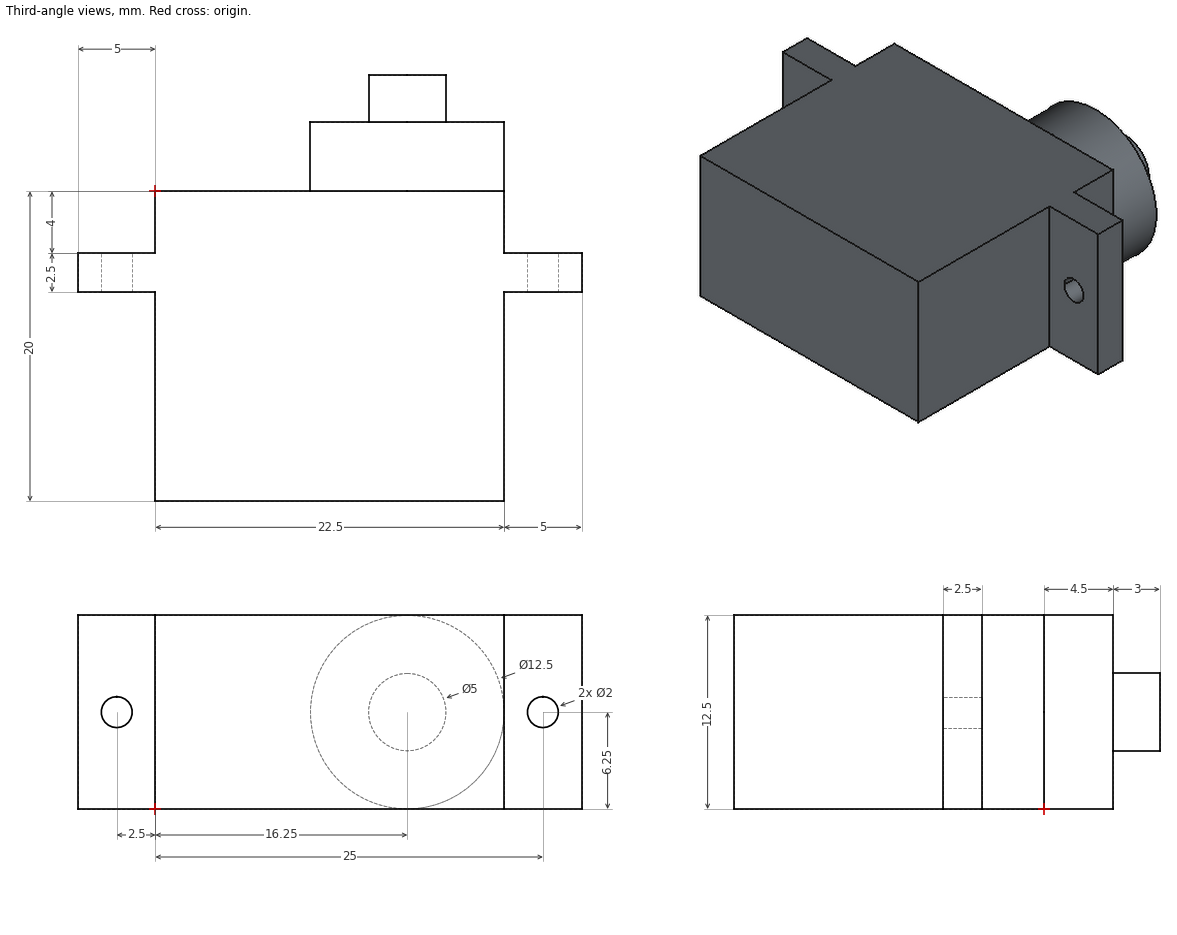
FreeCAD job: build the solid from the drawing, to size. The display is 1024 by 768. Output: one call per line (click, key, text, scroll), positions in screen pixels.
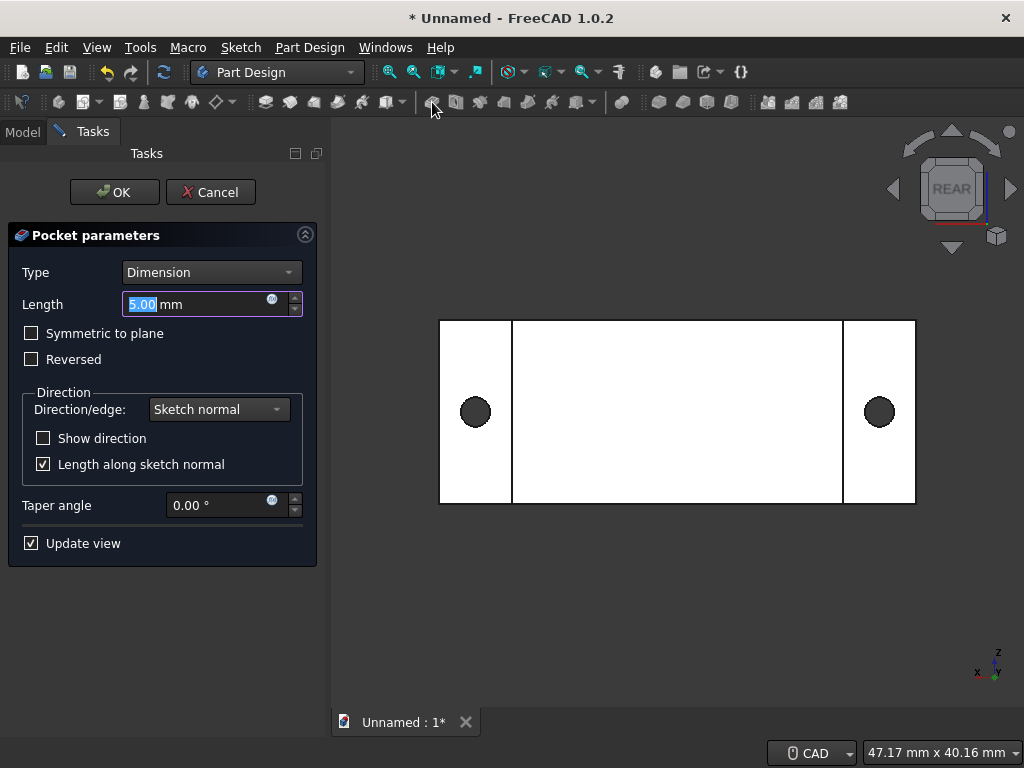
text(2.5)
key(Tab)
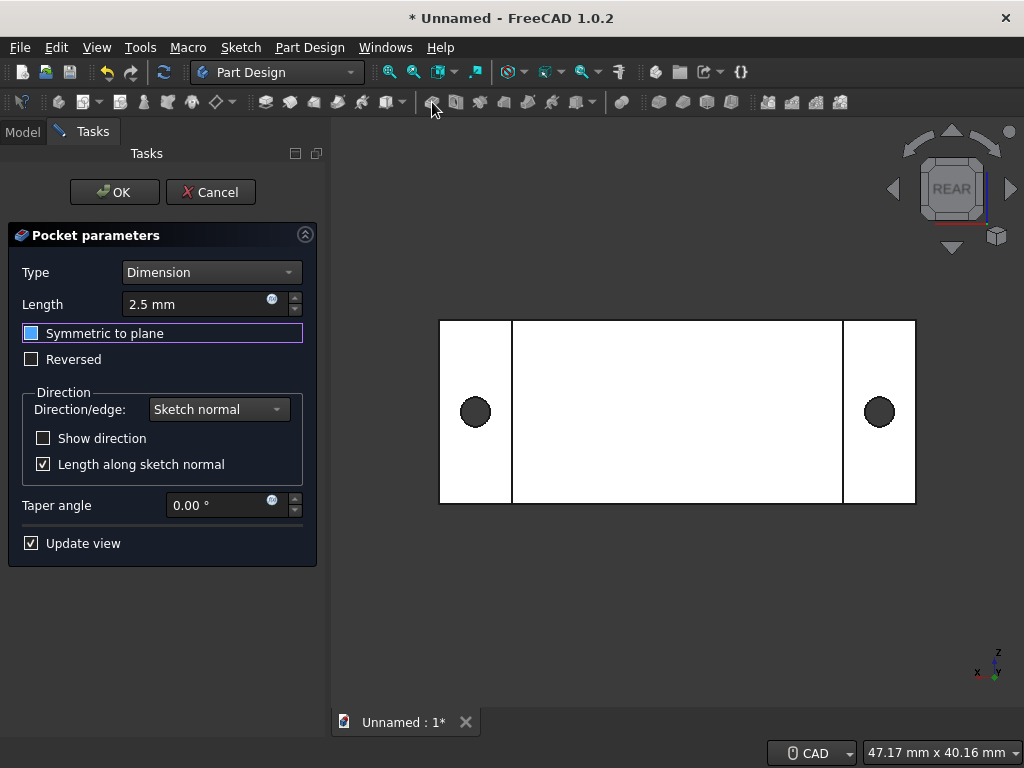
click(115, 192)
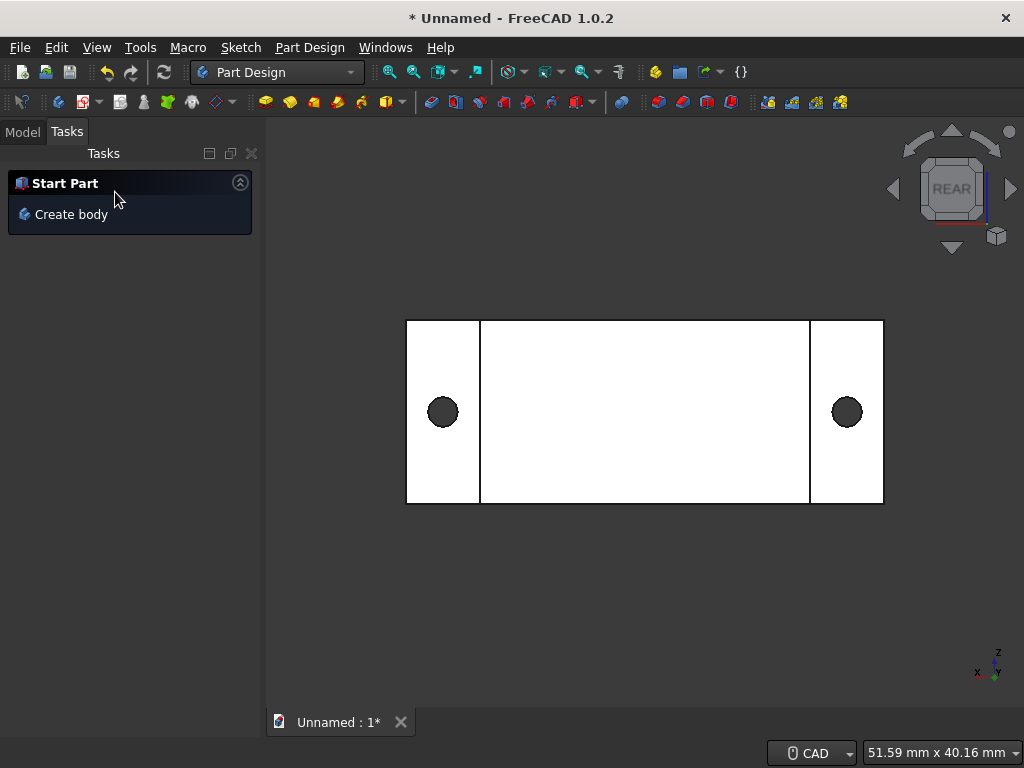
click(598, 411)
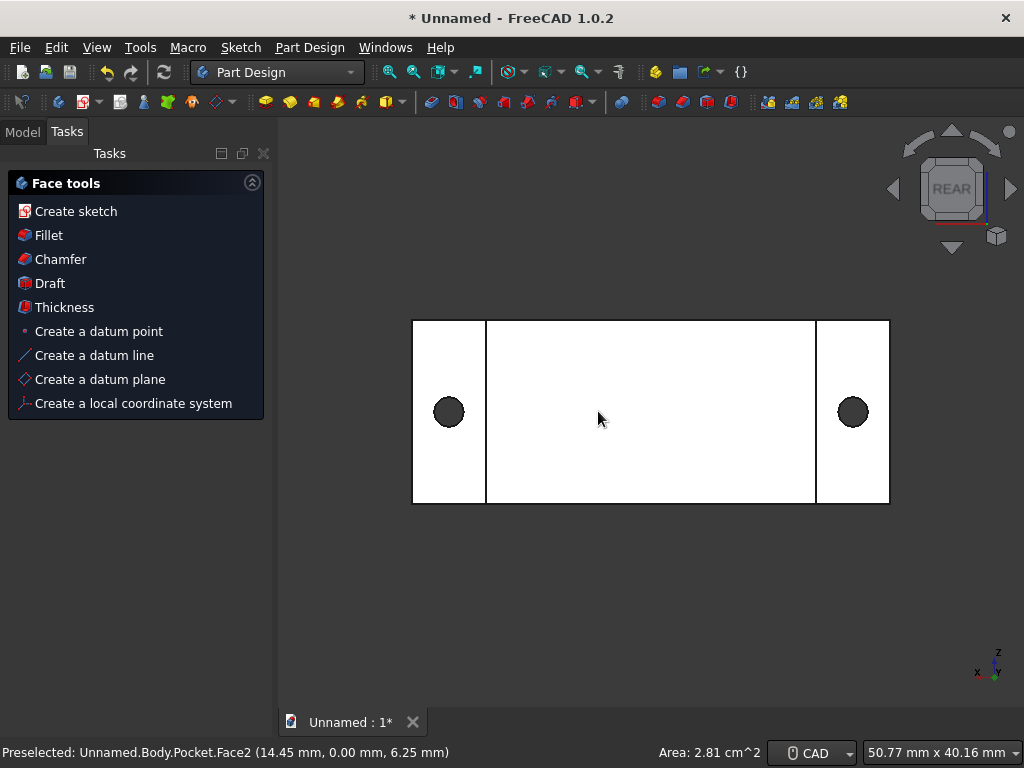
click(84, 102)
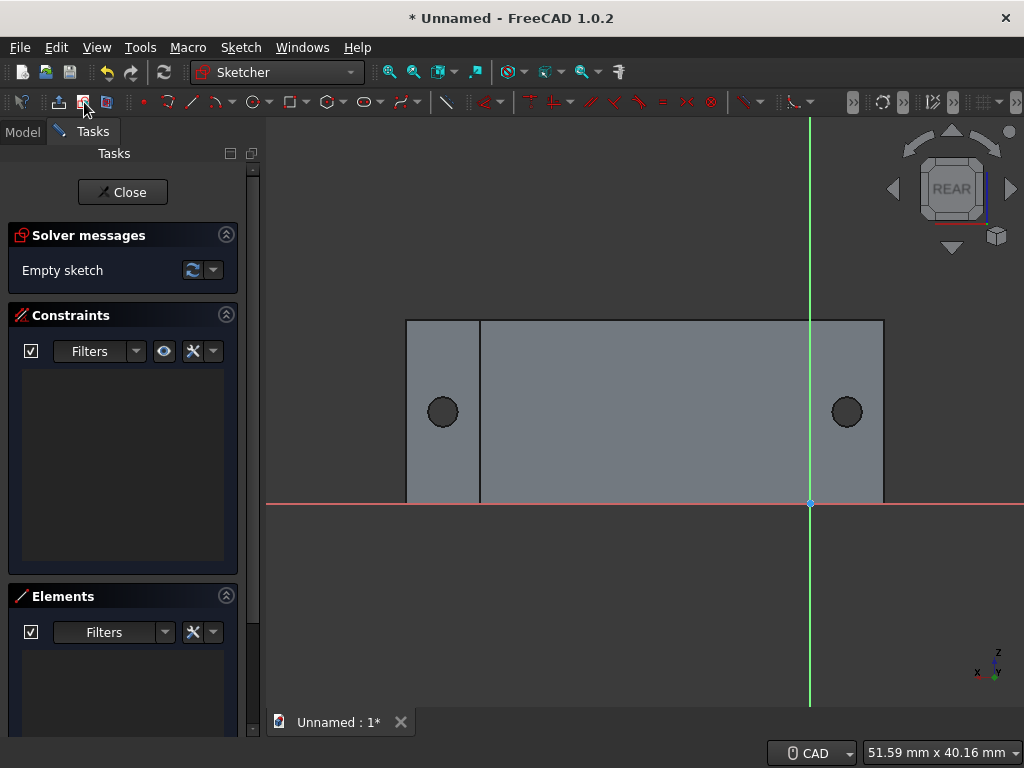
click(254, 102)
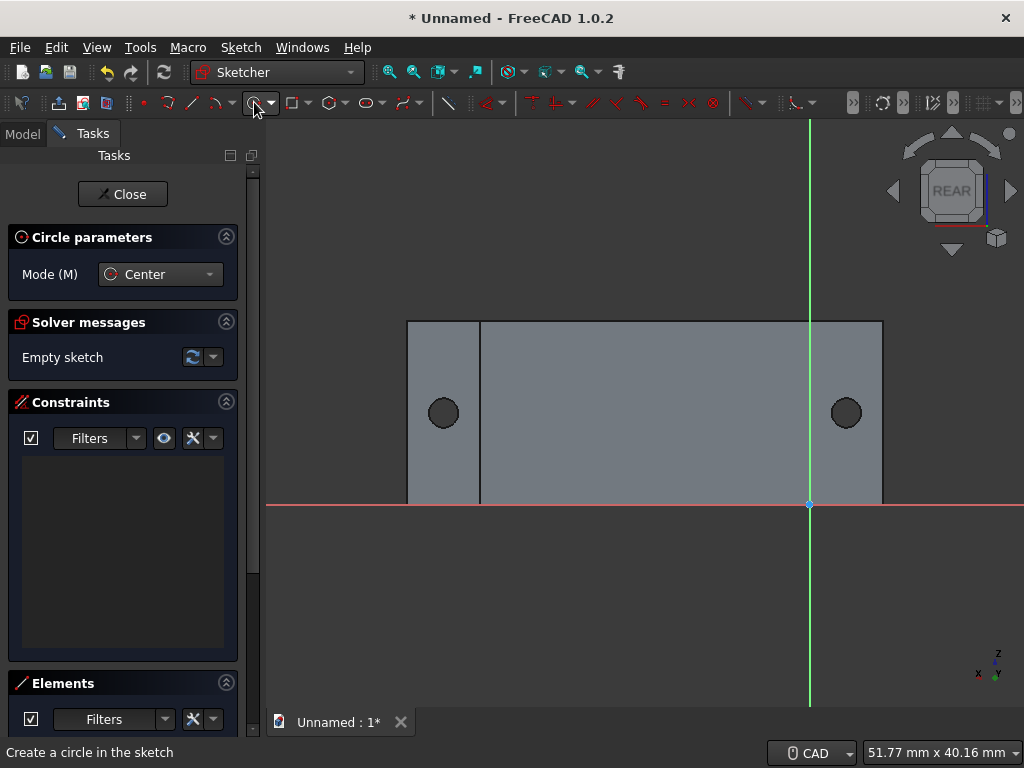
click(572, 413)
move(636, 348)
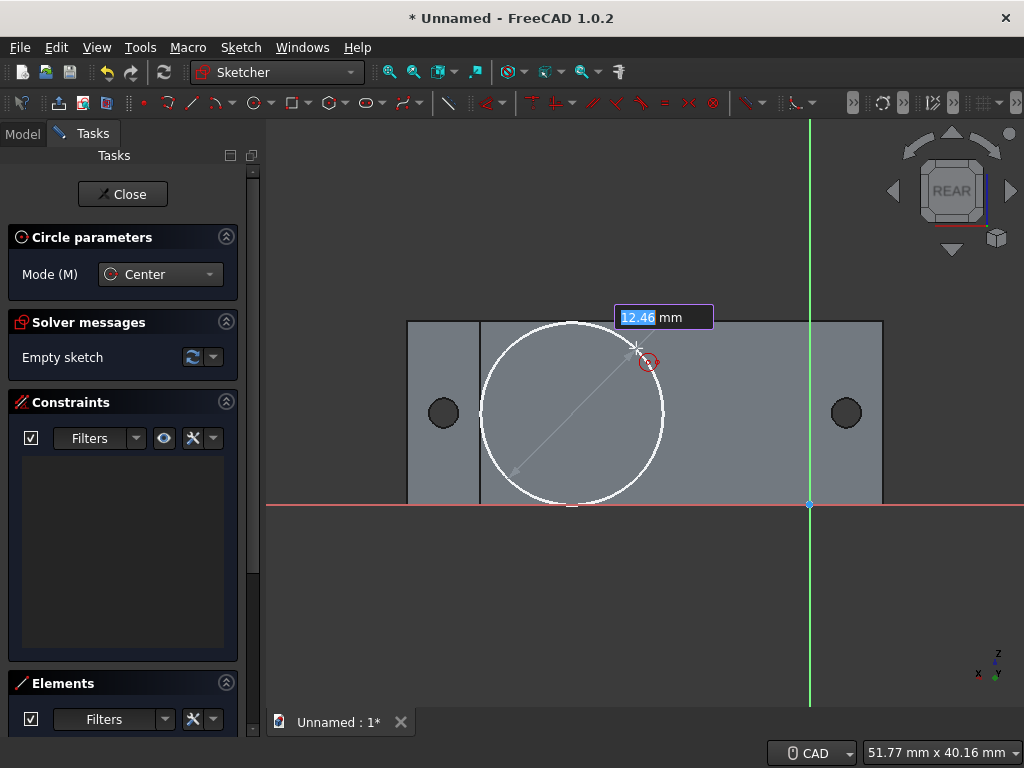
text(12.5)
key(Return)
key(Escape)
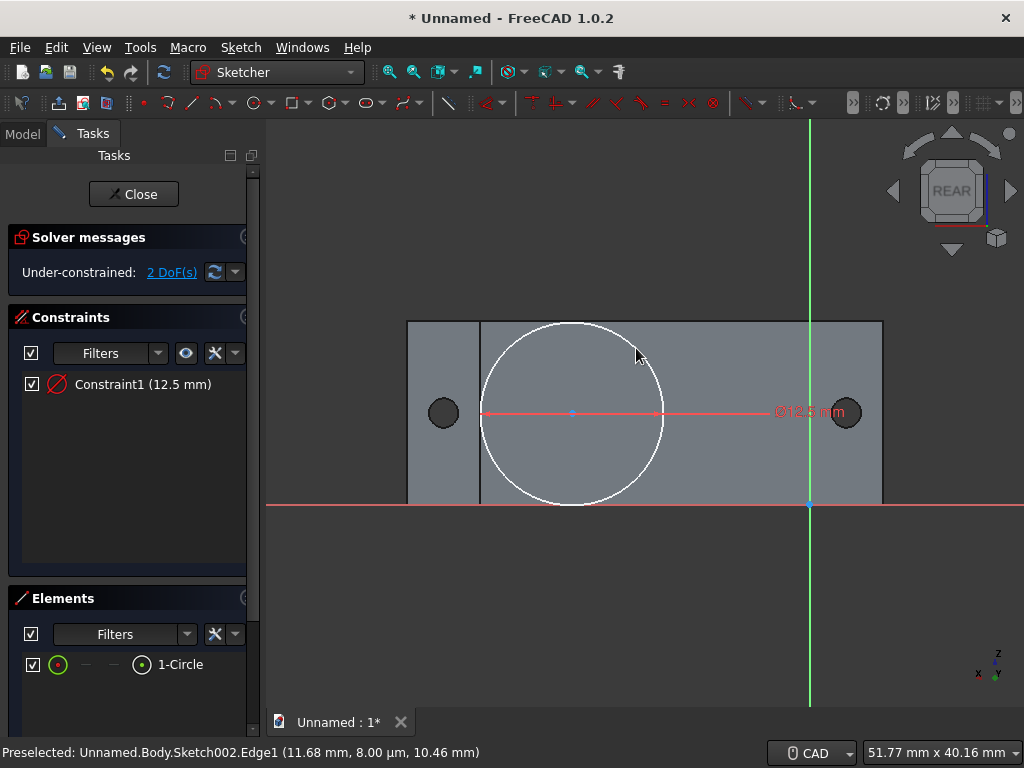
key(d)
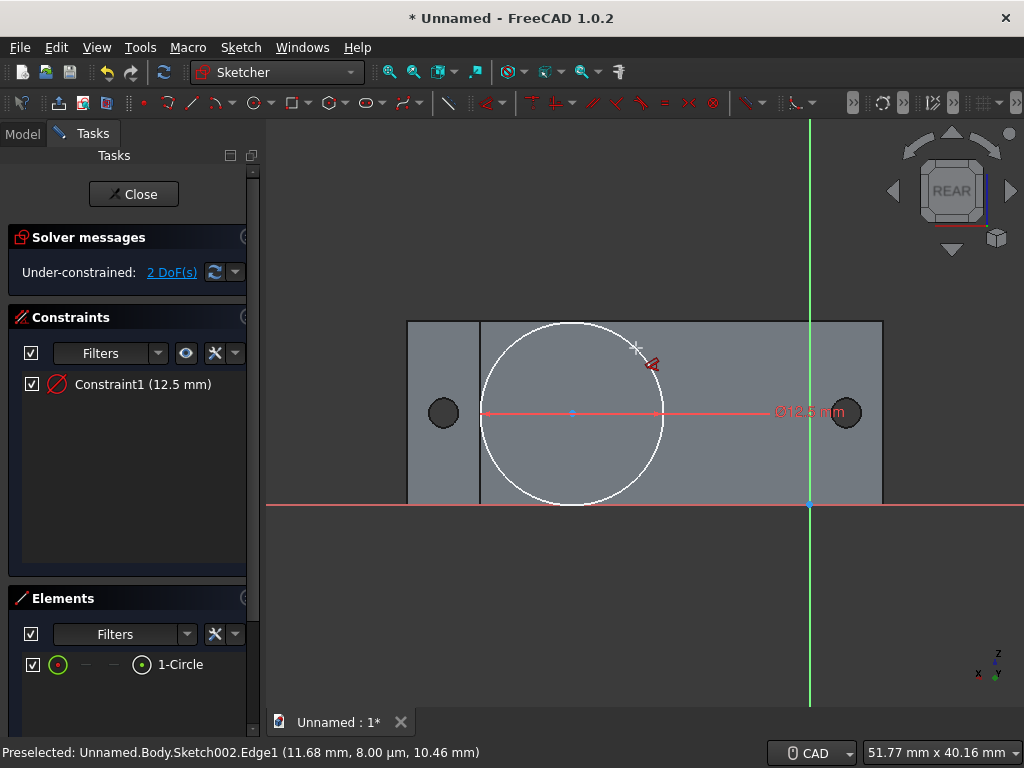
click(572, 414)
click(844, 459)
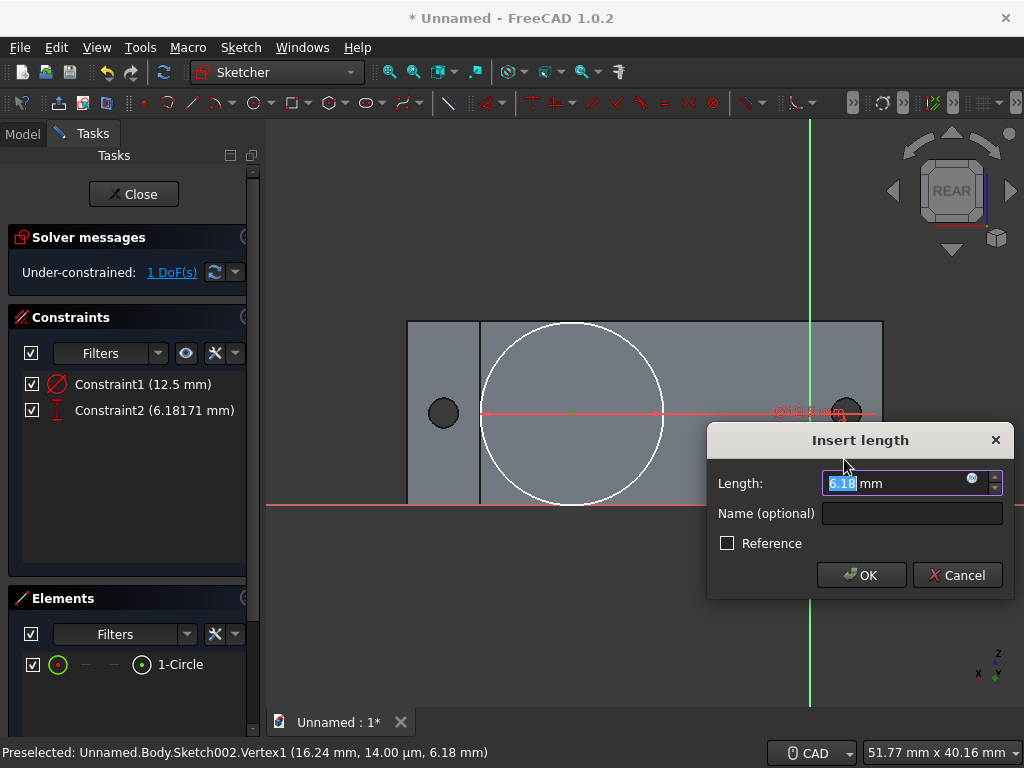
text(6.25)
key(Return)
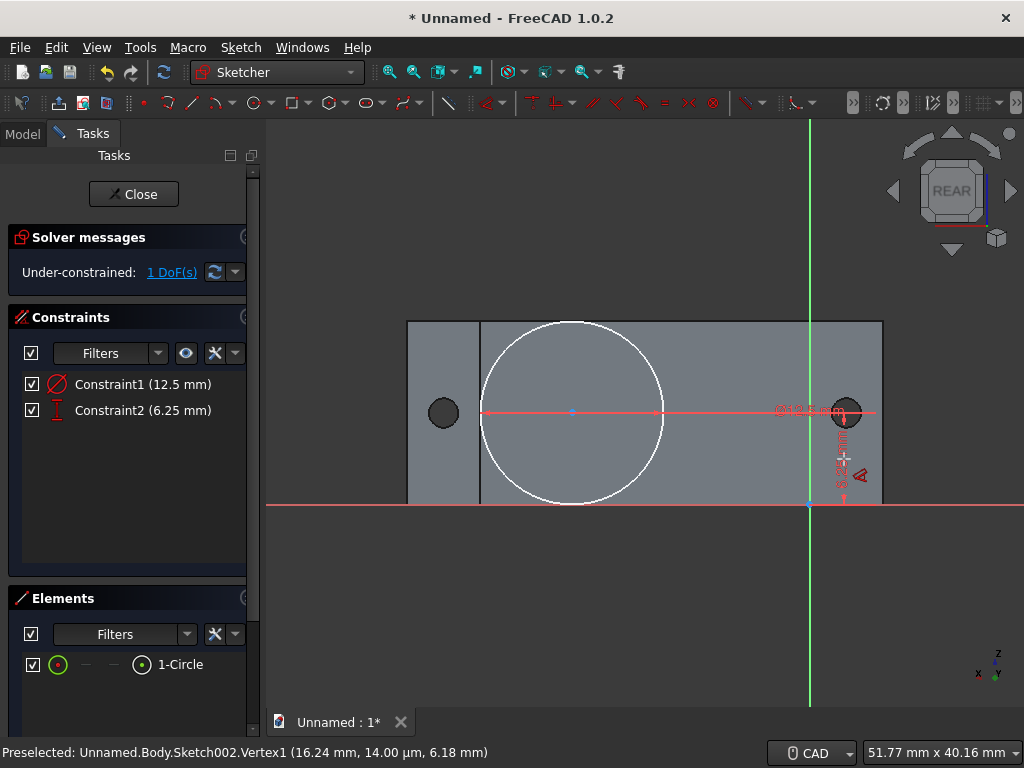
click(572, 413)
click(691, 539)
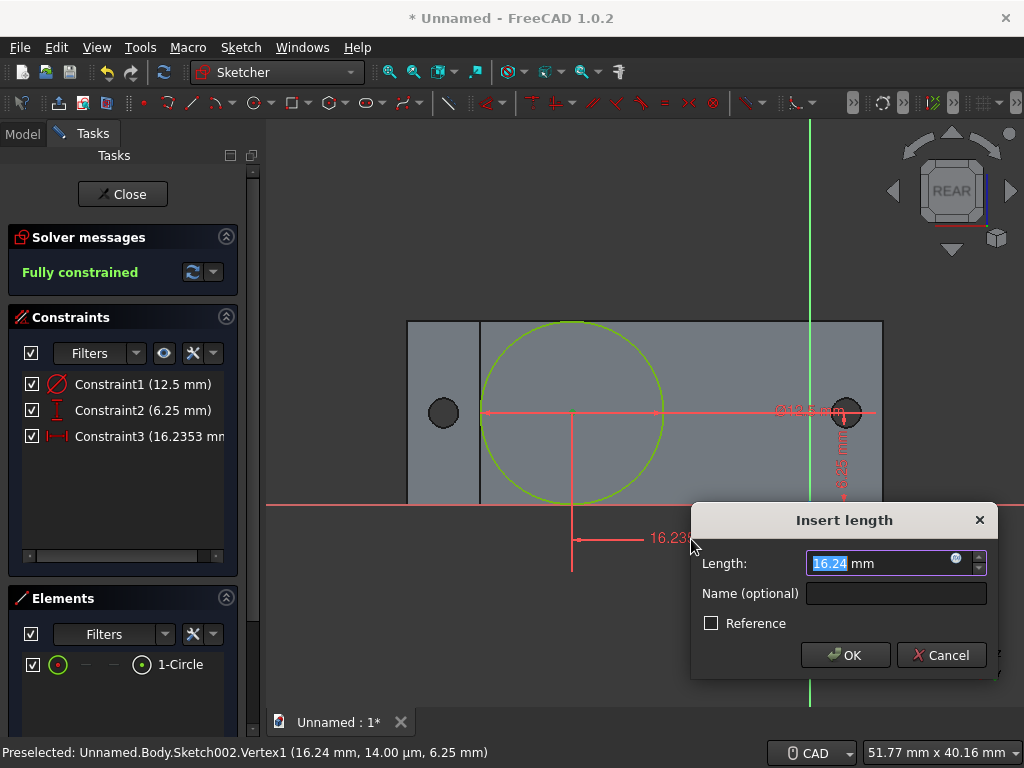
text(16.25)
key(Return)
key(Escape)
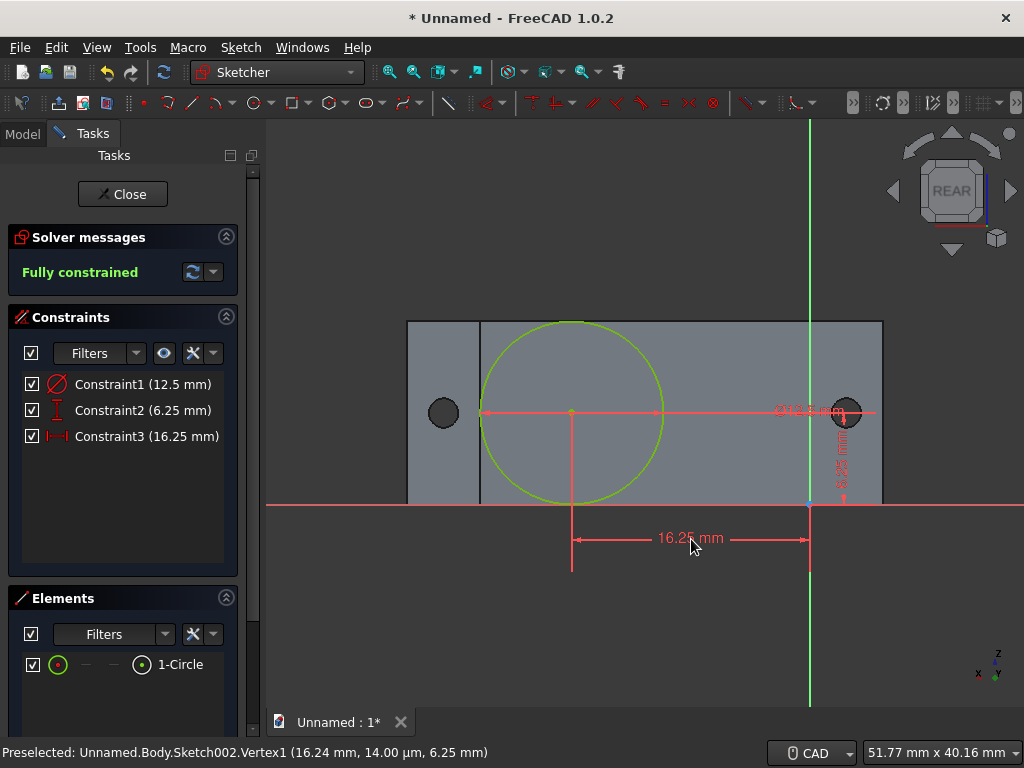
click(123, 194)